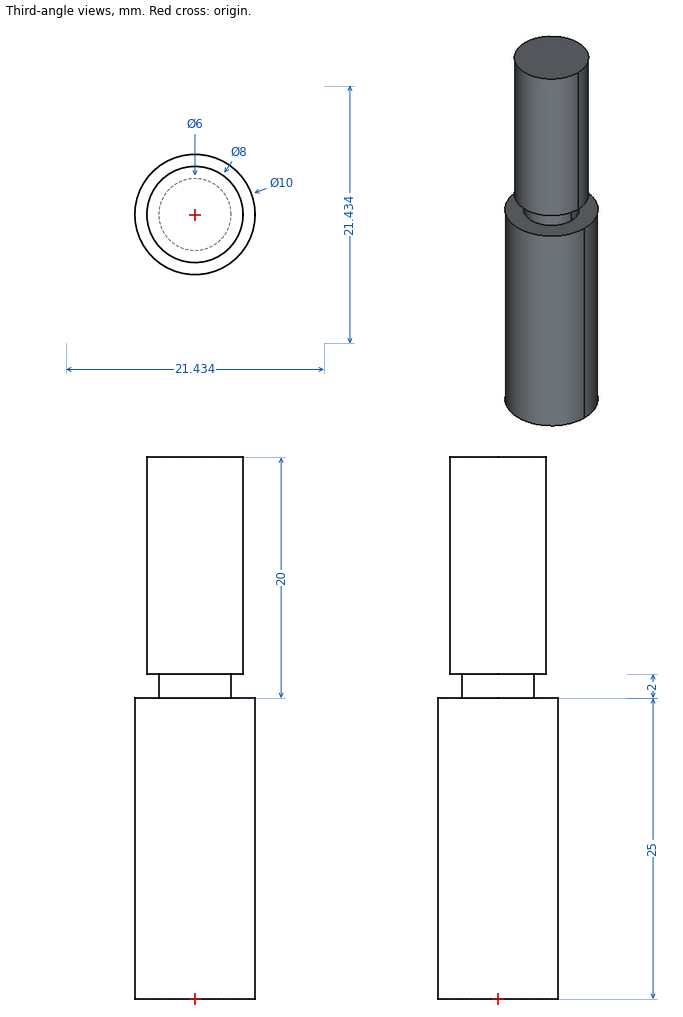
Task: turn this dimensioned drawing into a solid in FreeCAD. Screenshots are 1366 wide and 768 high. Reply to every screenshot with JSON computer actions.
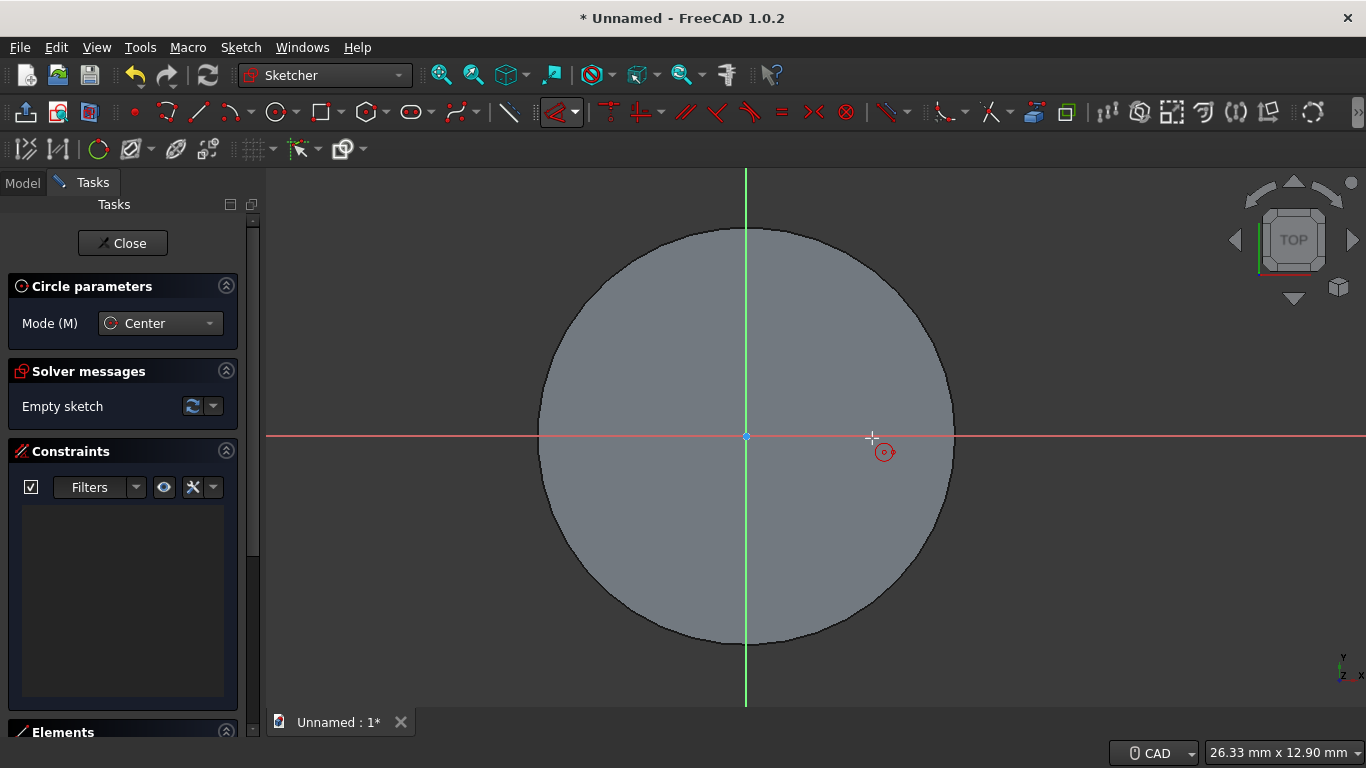
{"action": "left_click", "coordinate": [746, 436]}
{"action": "left_click", "coordinate": [865, 318]}
{"action": "key", "text": "Escape"}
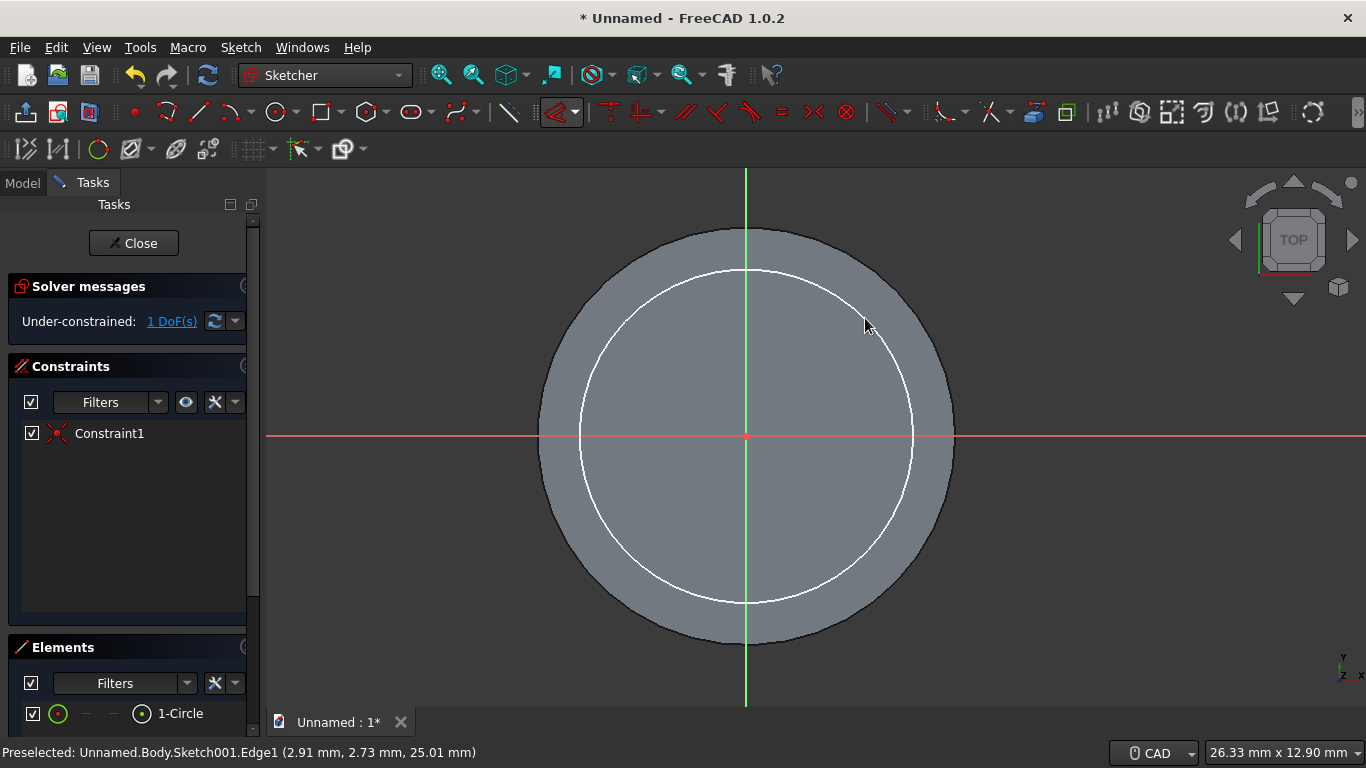
{"action": "left_click", "coordinate": [864, 318]}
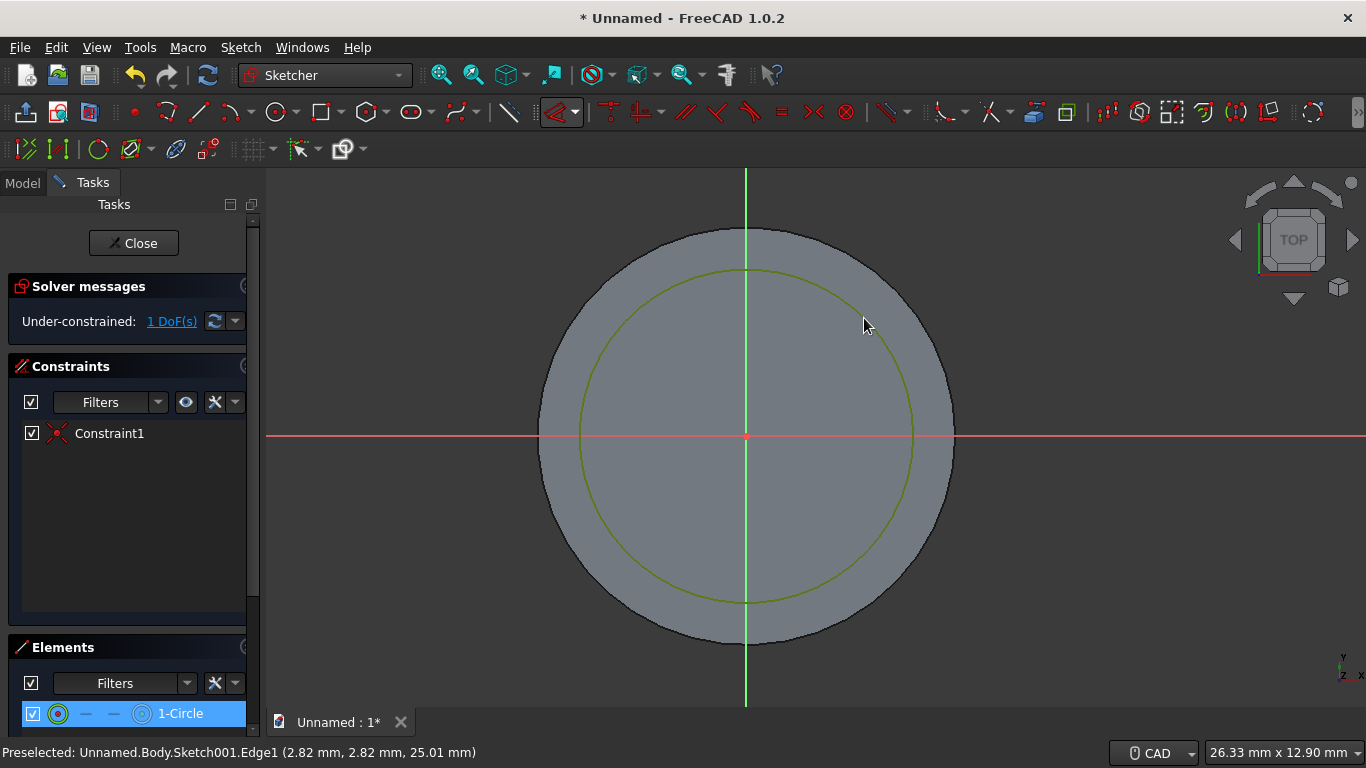
{"action": "left_click", "coordinate": [578, 112]}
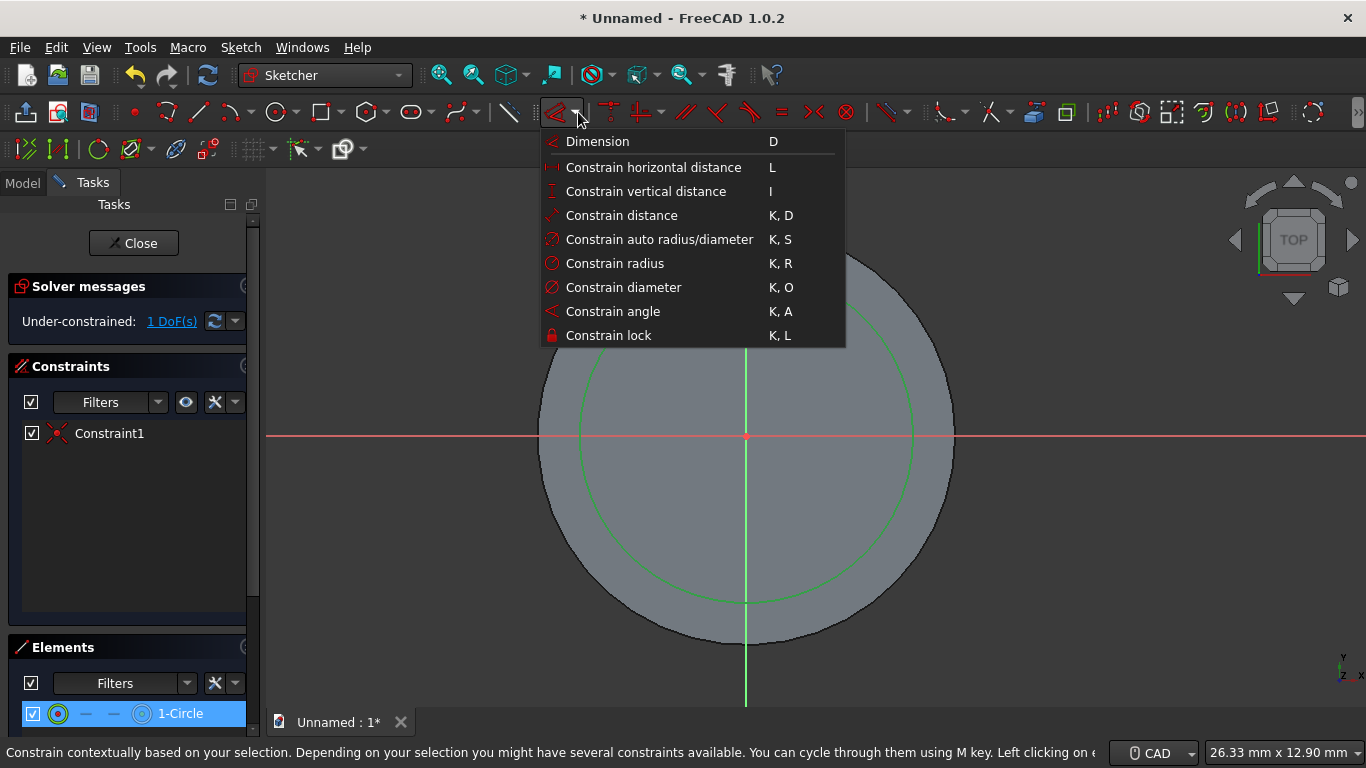
{"action": "left_click", "coordinate": [693, 287]}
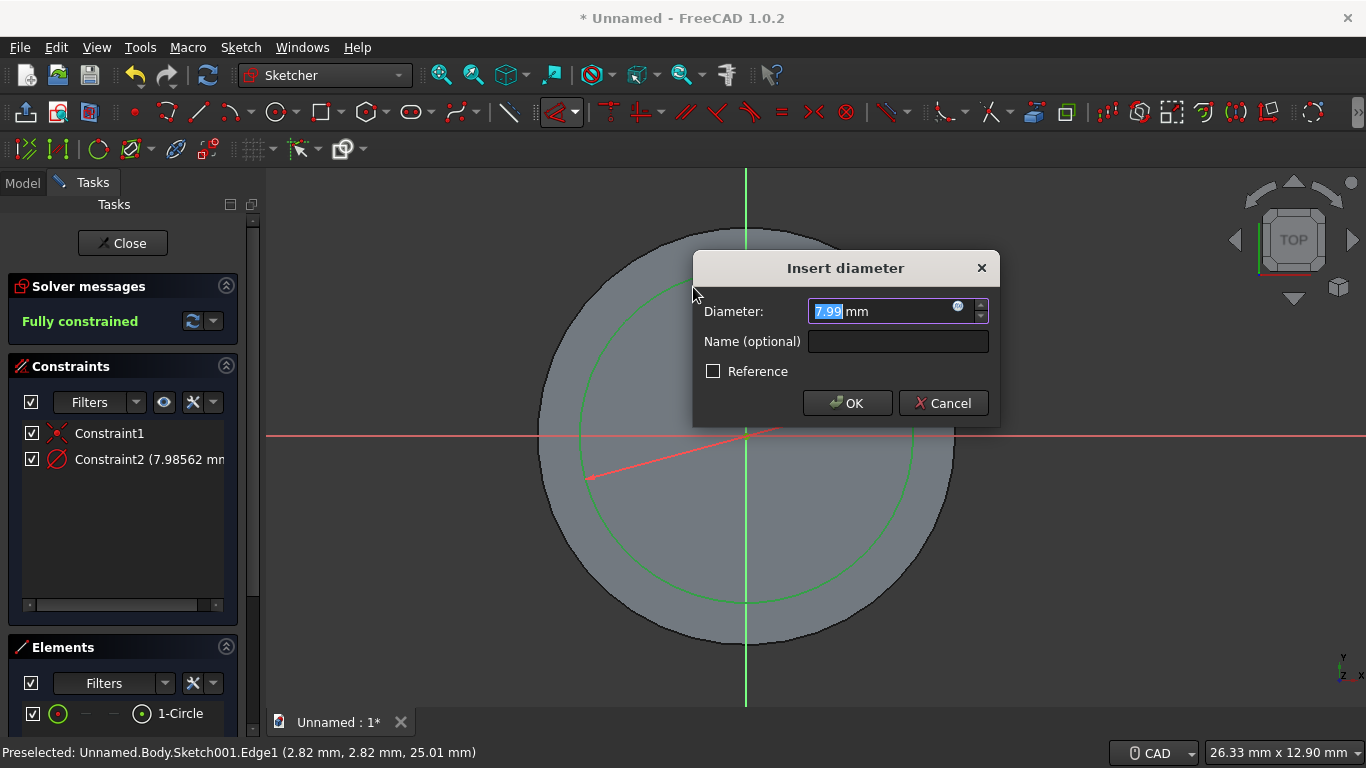
{"action": "type", "text": "8"}
{"action": "key", "text": "Return"}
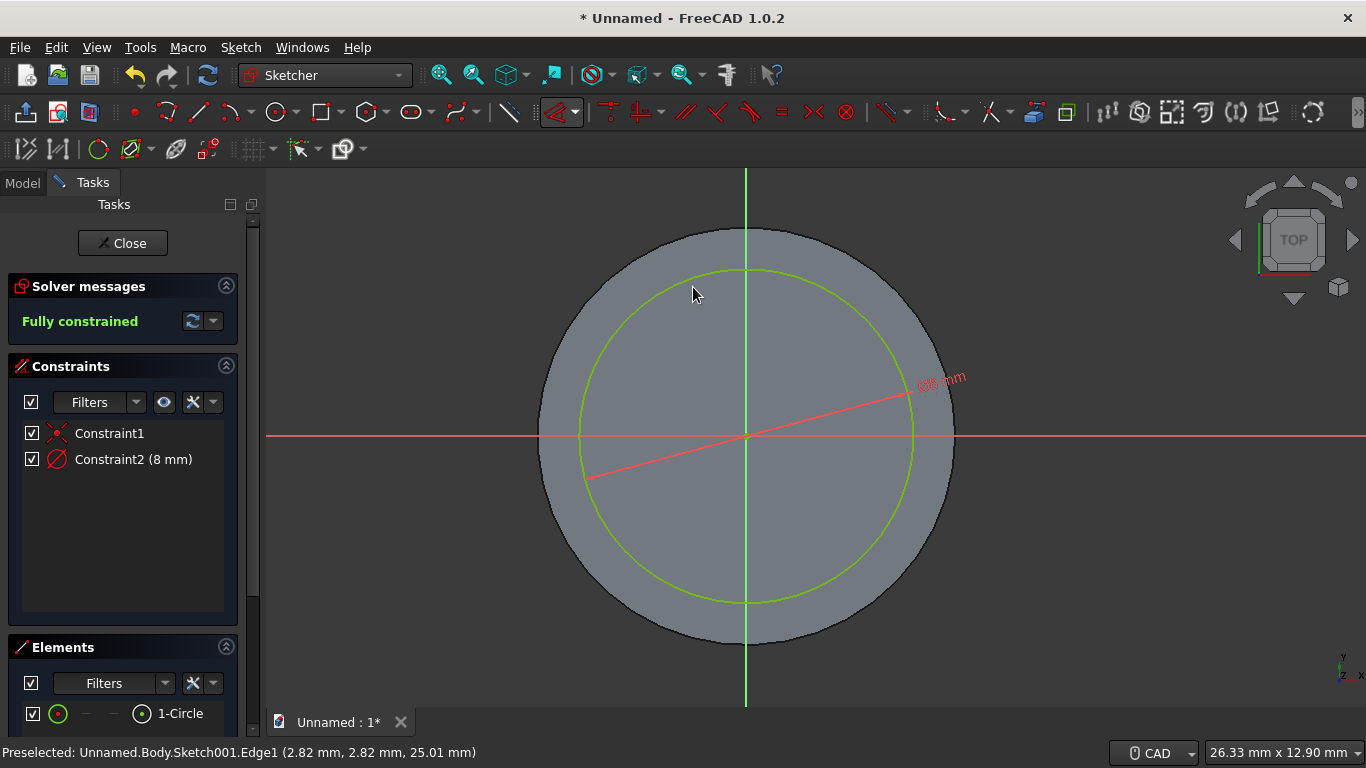
{"action": "left_click", "coordinate": [123, 243]}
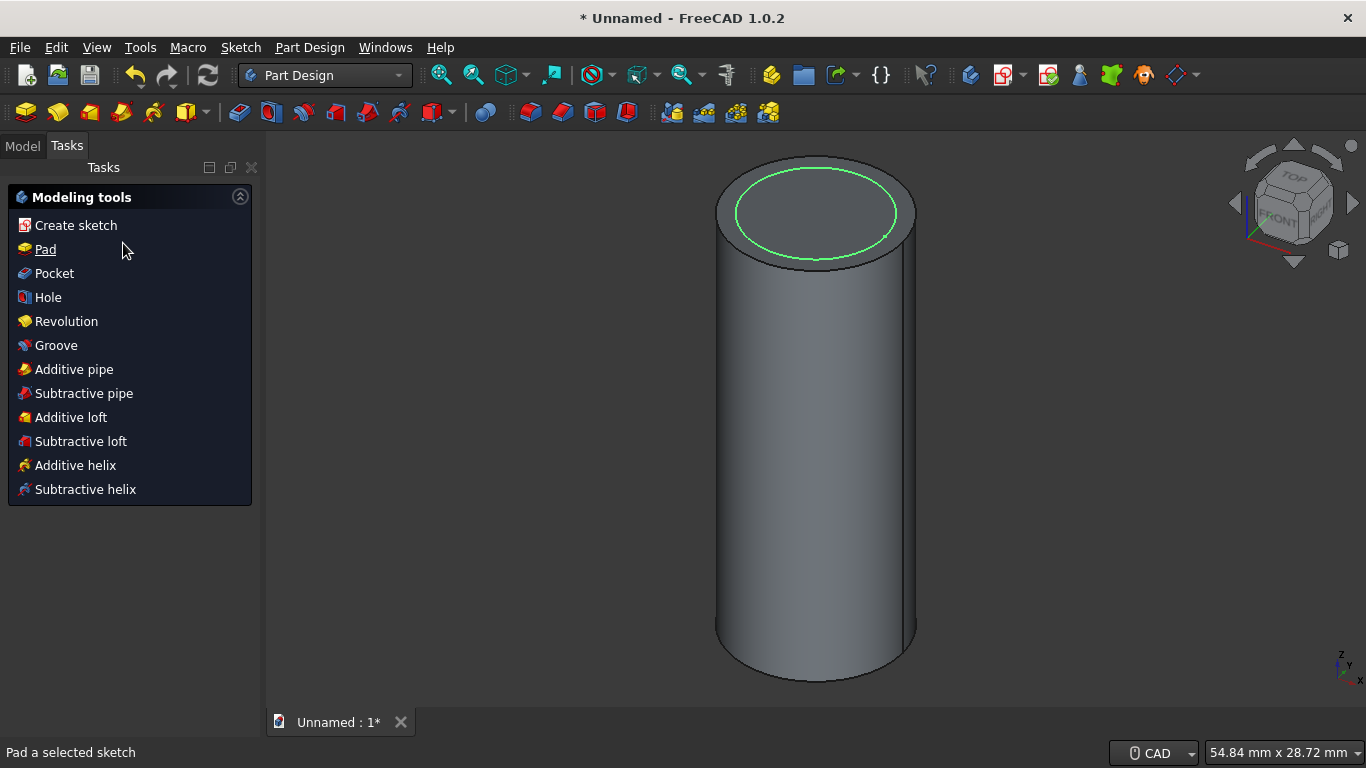
{"action": "left_click", "coordinate": [26, 112]}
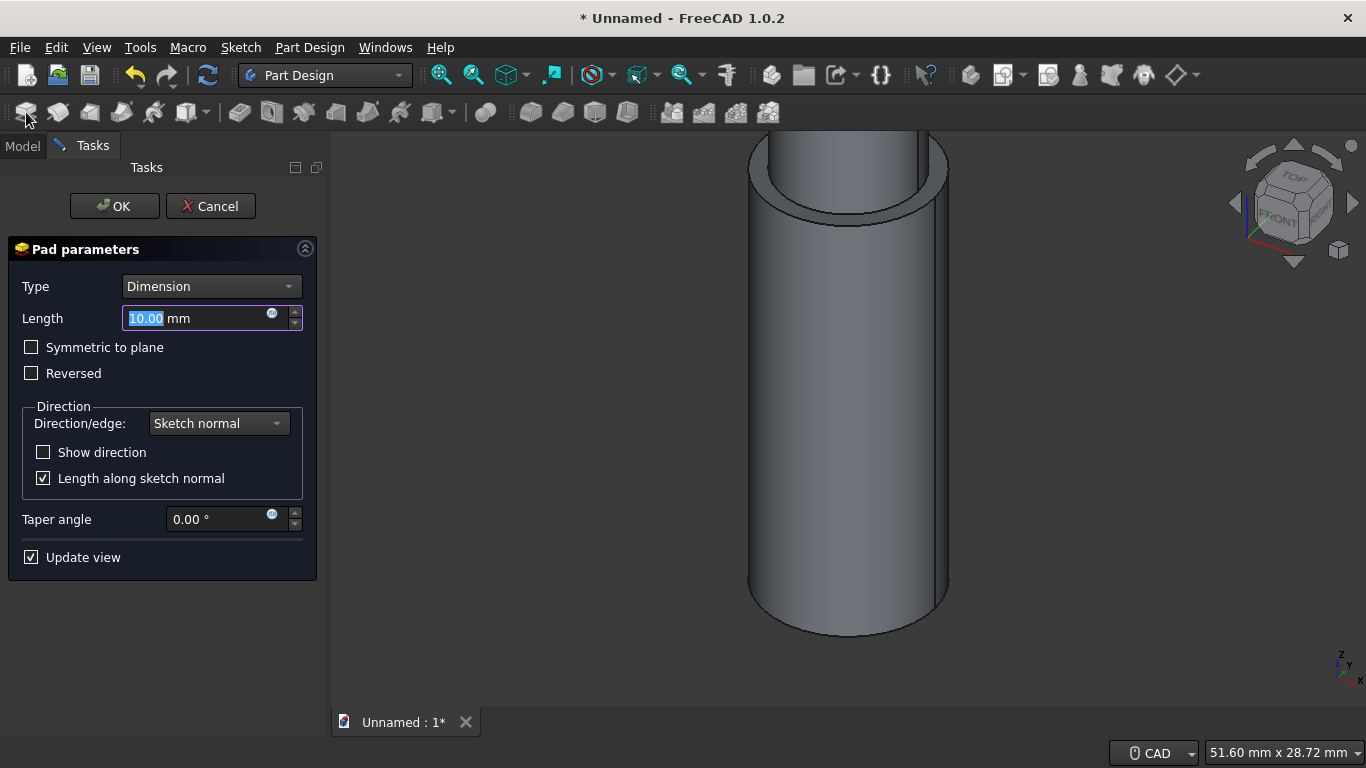
{"action": "type", "text": "20"}
{"action": "key", "text": "Tab"}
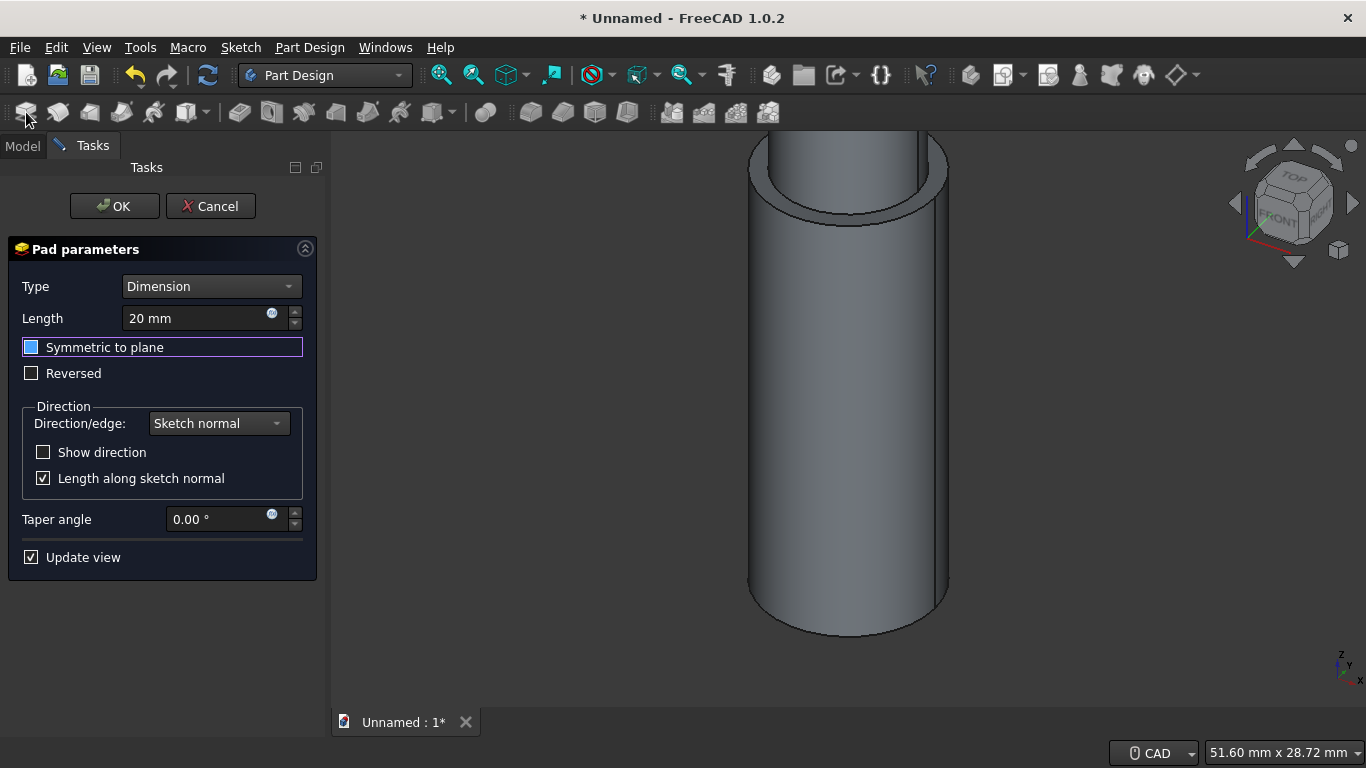
{"action": "left_click", "coordinate": [115, 206]}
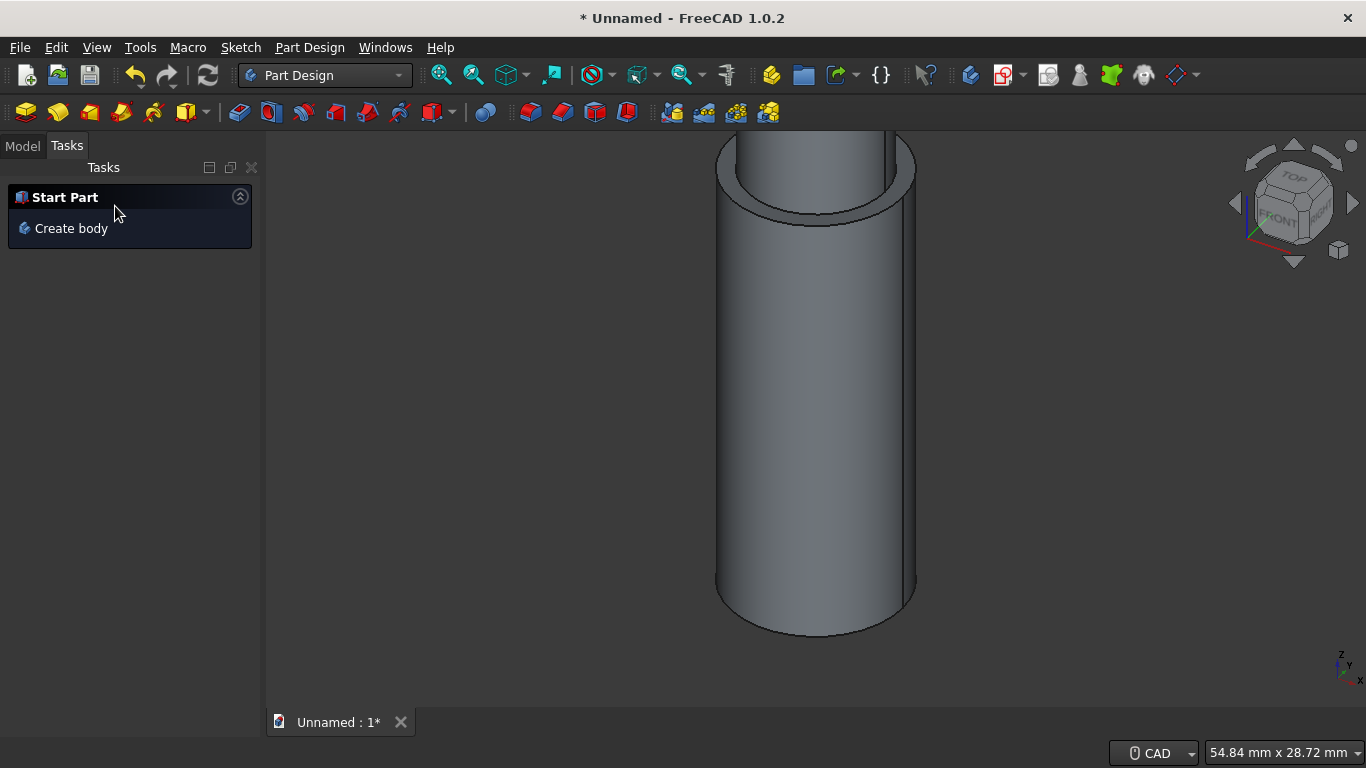
{"action": "key", "text": "v f"}